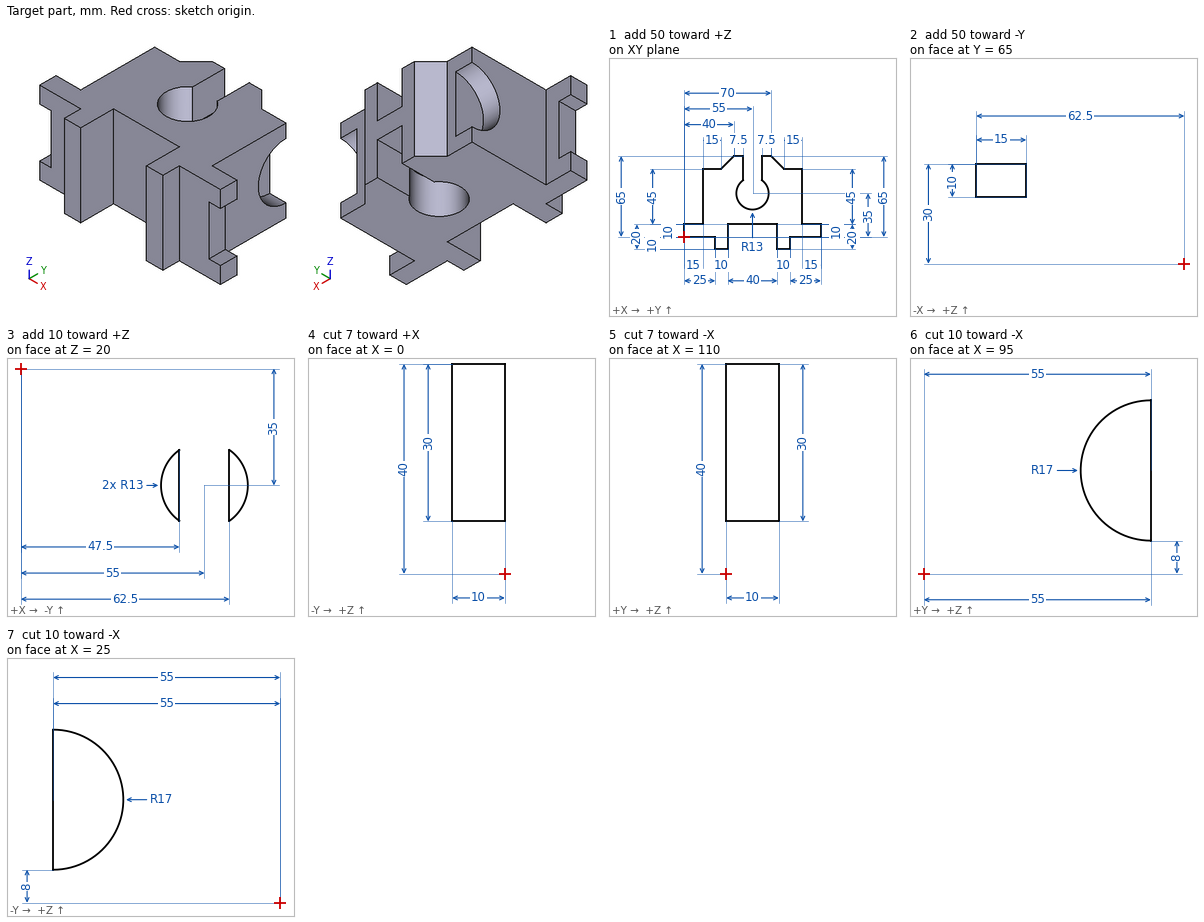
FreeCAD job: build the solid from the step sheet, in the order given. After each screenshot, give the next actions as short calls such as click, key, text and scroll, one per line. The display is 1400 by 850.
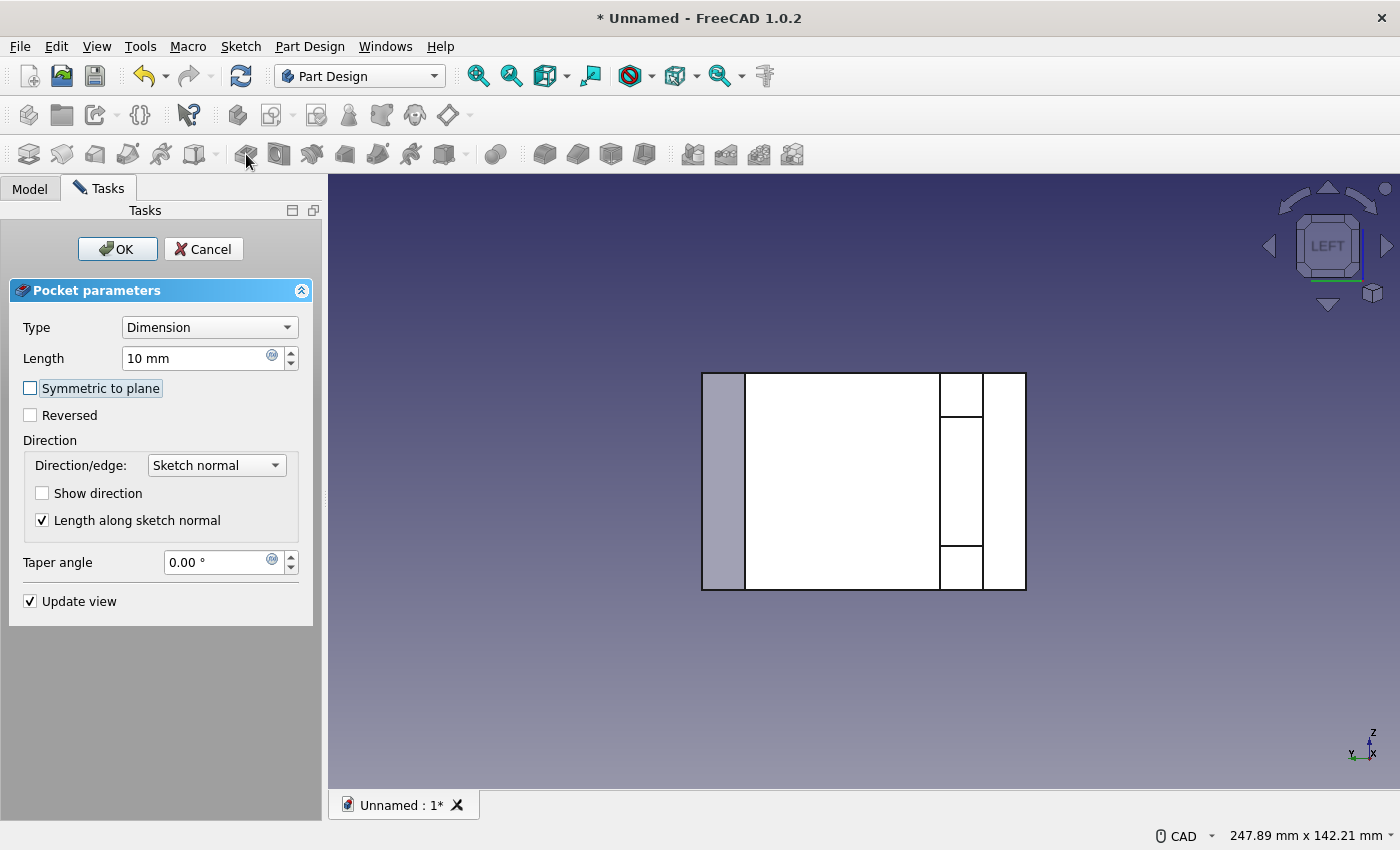
click(31, 415)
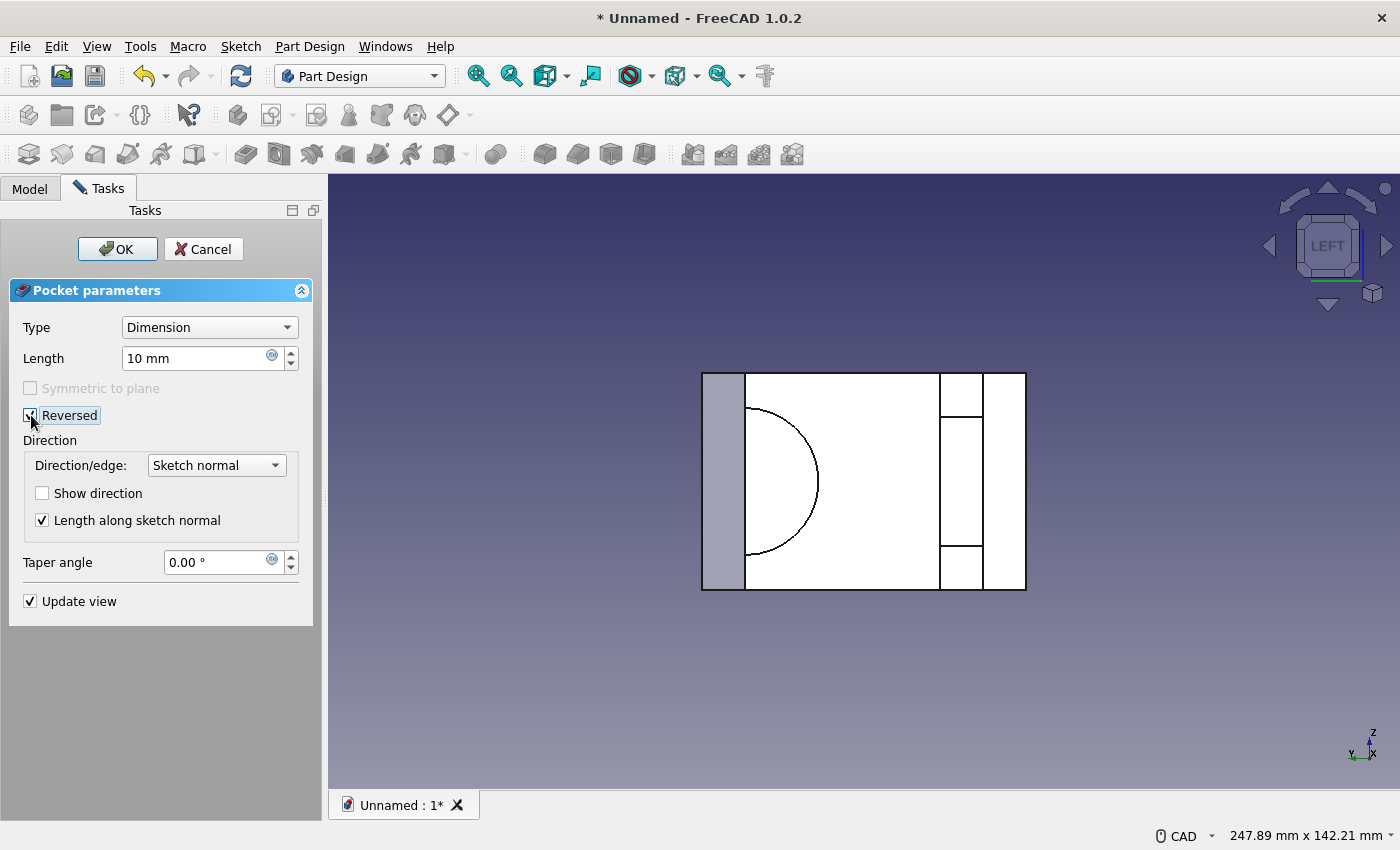
click(118, 249)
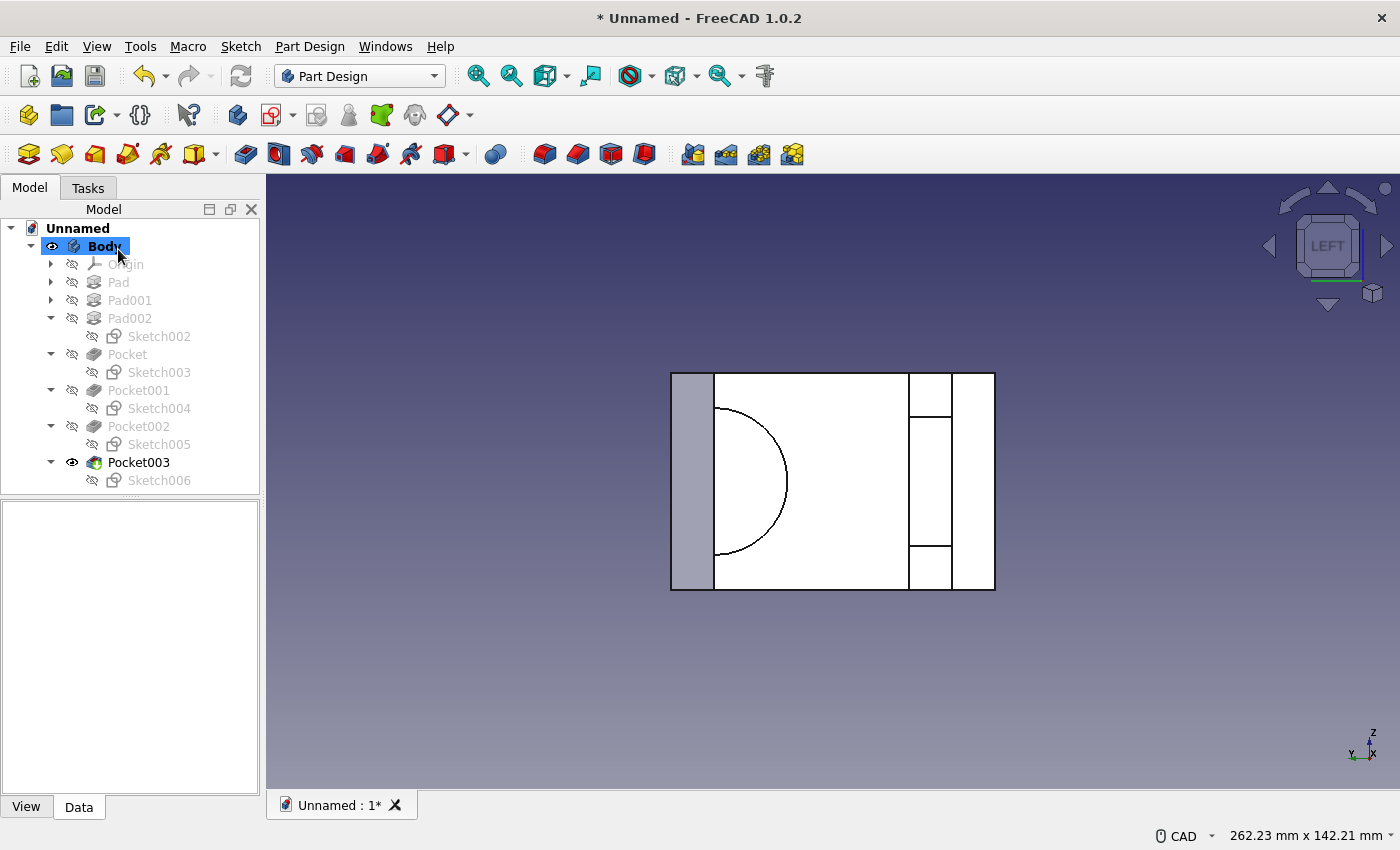
key(0)